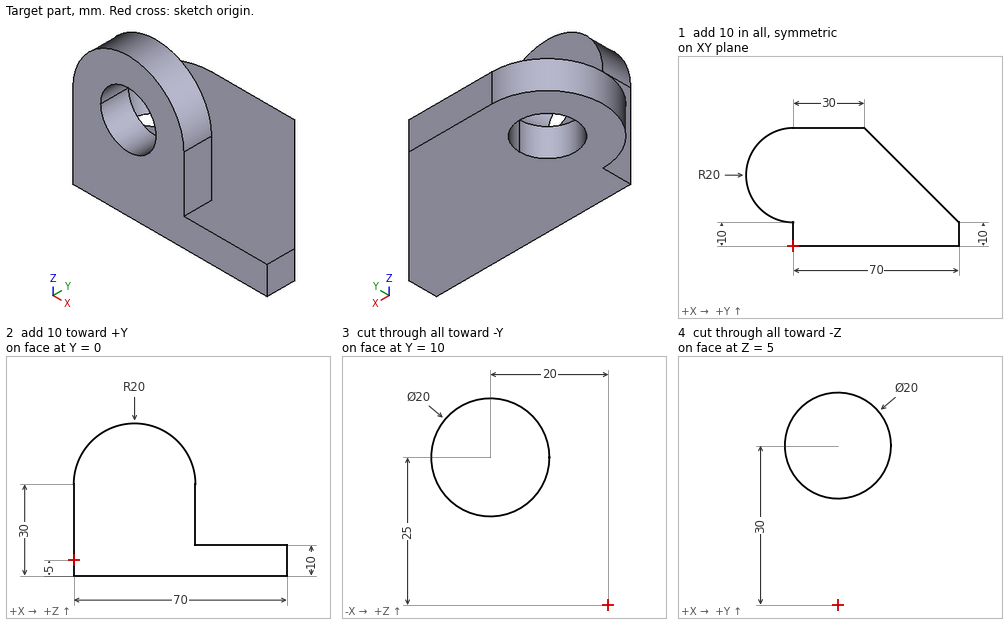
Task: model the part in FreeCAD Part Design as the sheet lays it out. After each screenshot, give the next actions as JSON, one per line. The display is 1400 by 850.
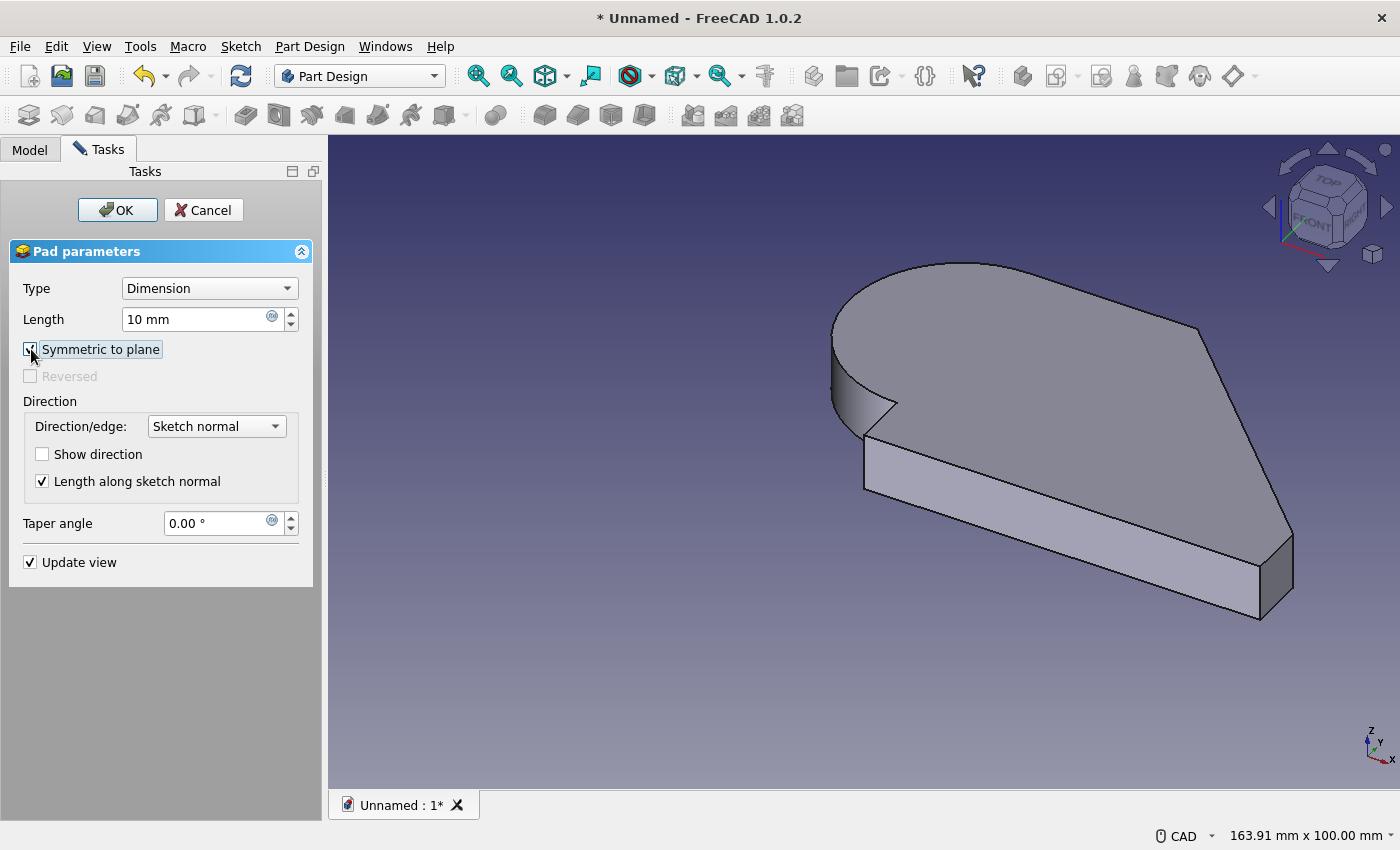
{"action": "left_click", "coordinate": [118, 210]}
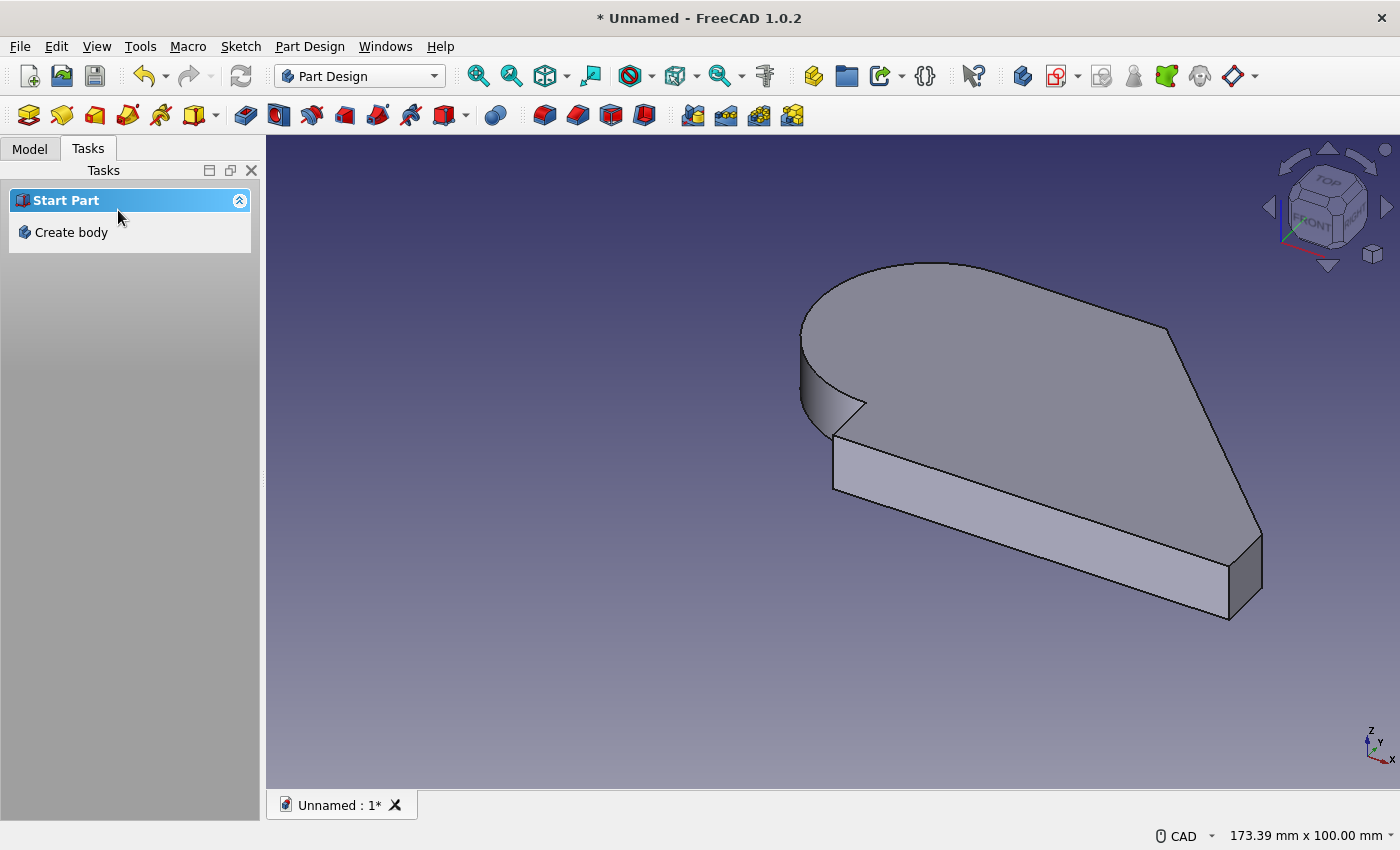
{"action": "left_click", "coordinate": [1201, 583]}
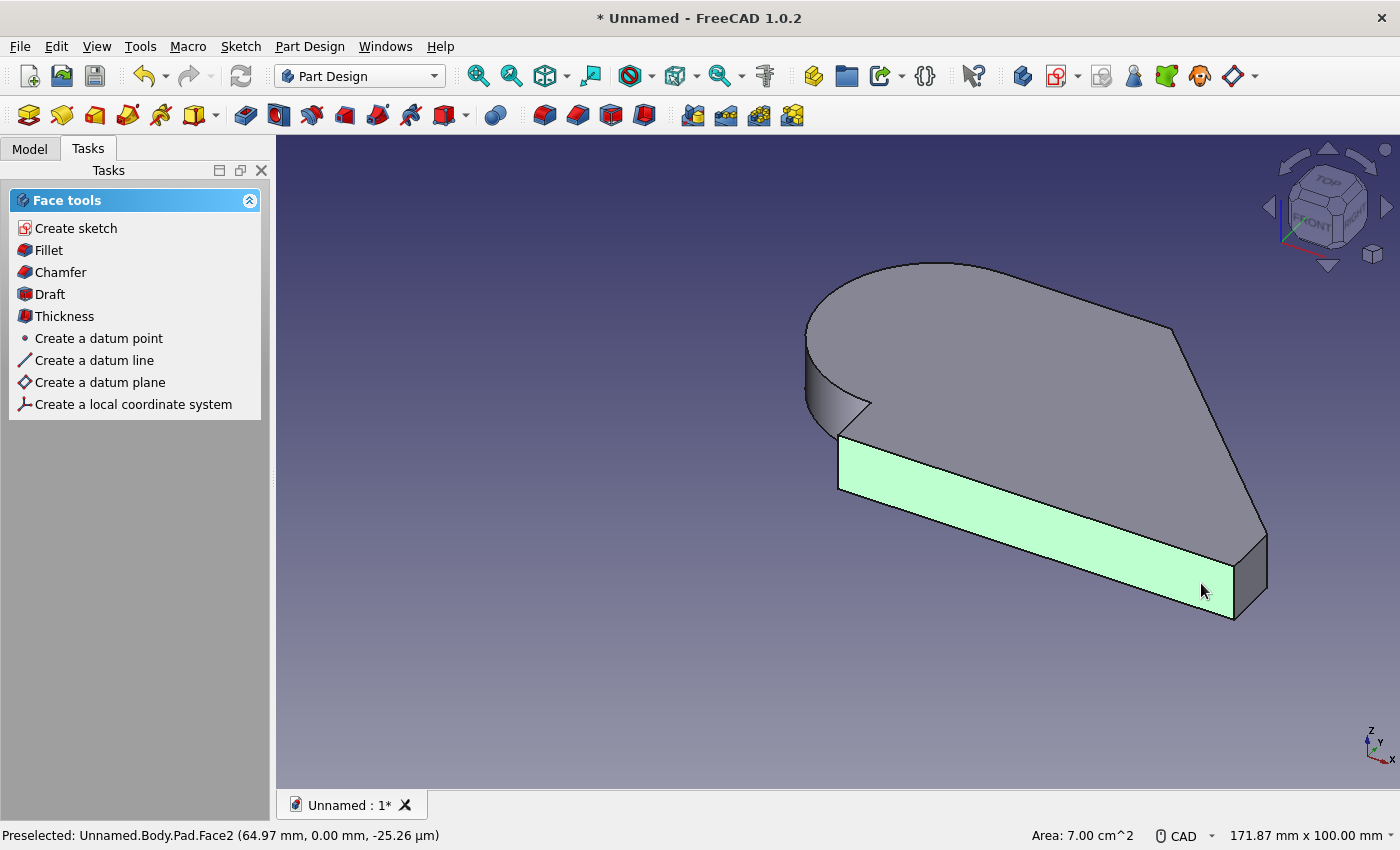
{"action": "left_click", "coordinate": [1056, 76]}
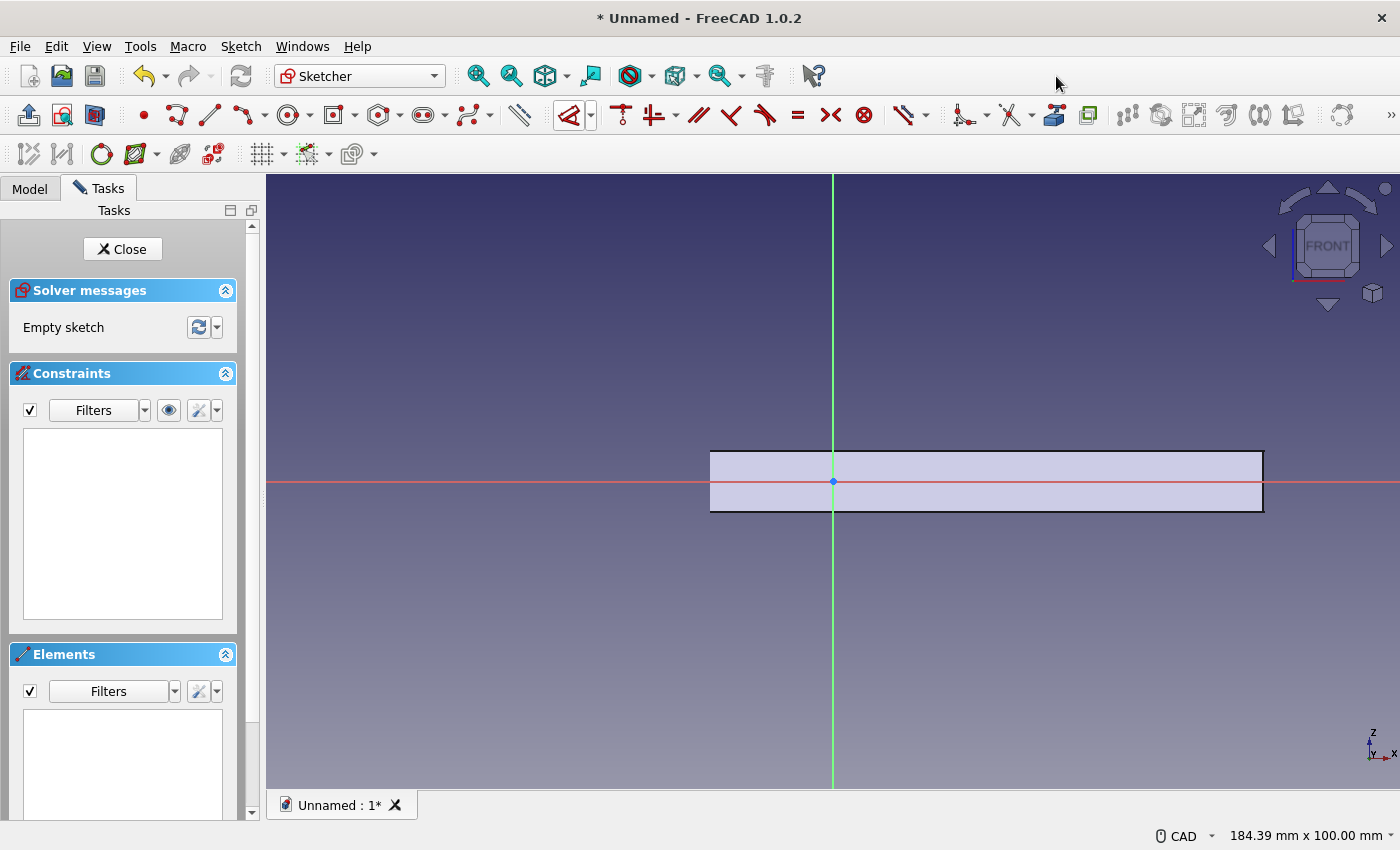
{"action": "scroll", "coordinate": [294, 761], "scroll_direction": "down", "scroll_amount": 1}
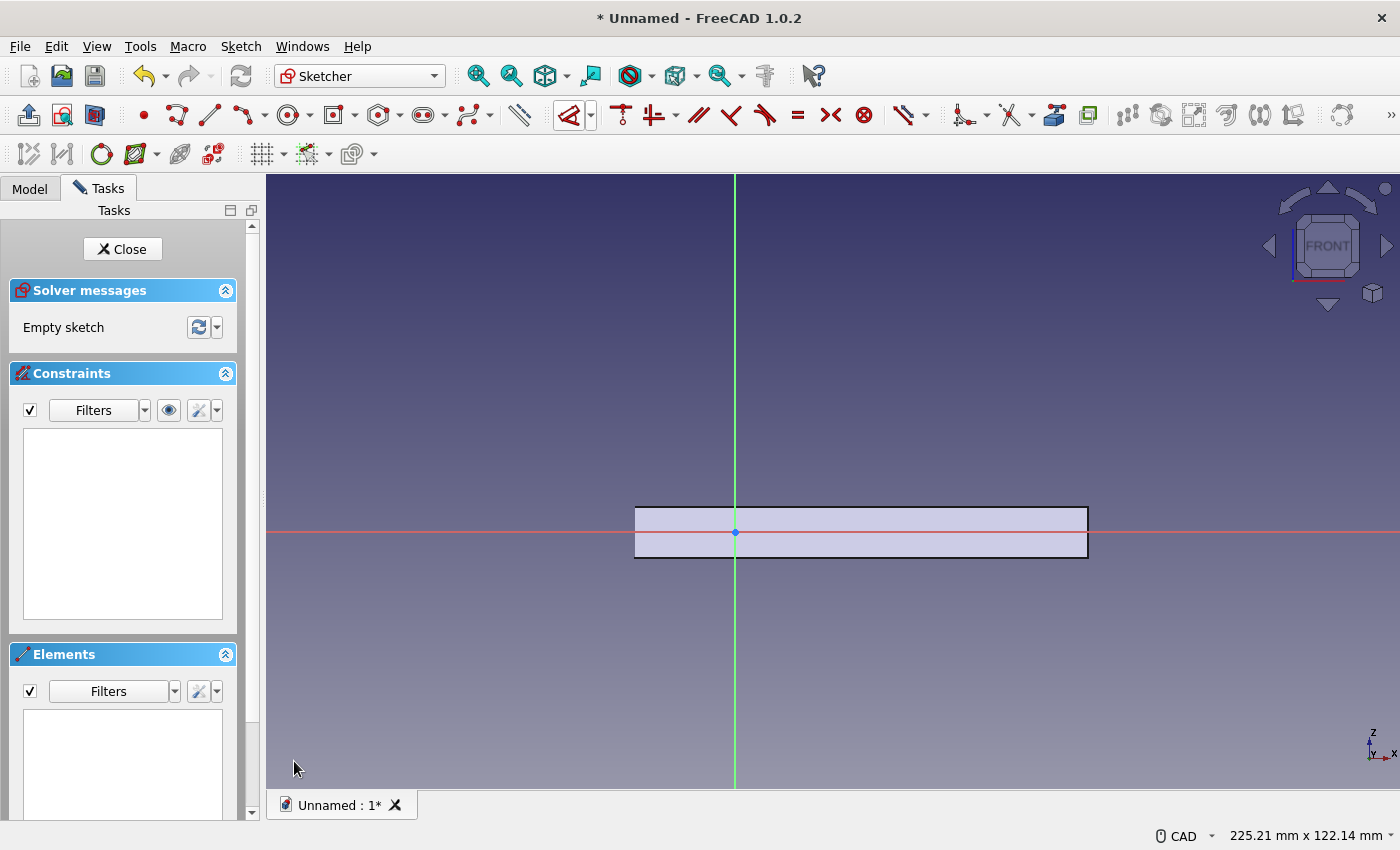
{"action": "scroll", "coordinate": [1210, 330], "scroll_direction": "up", "scroll_amount": 2}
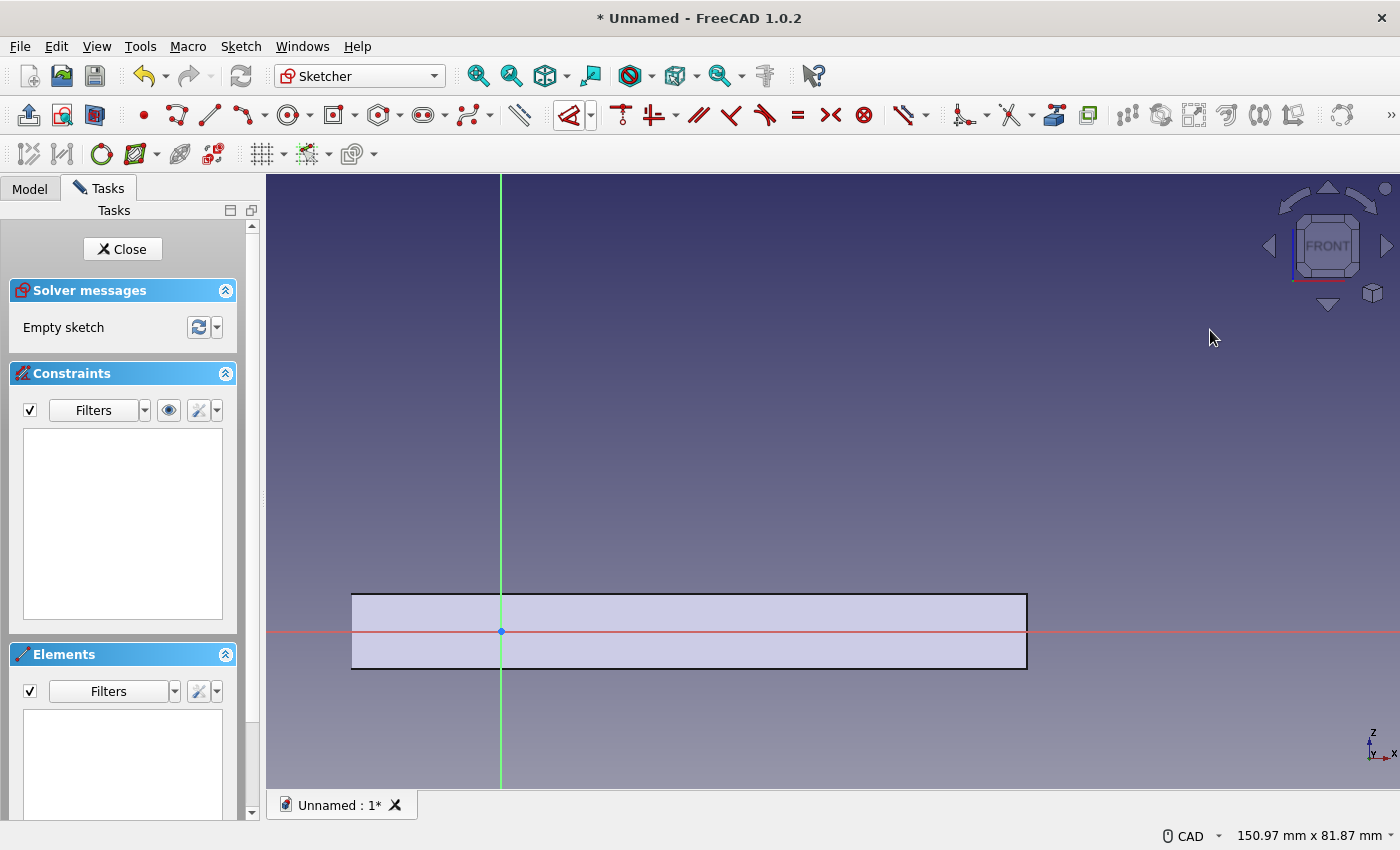
{"action": "left_click", "coordinate": [177, 116]}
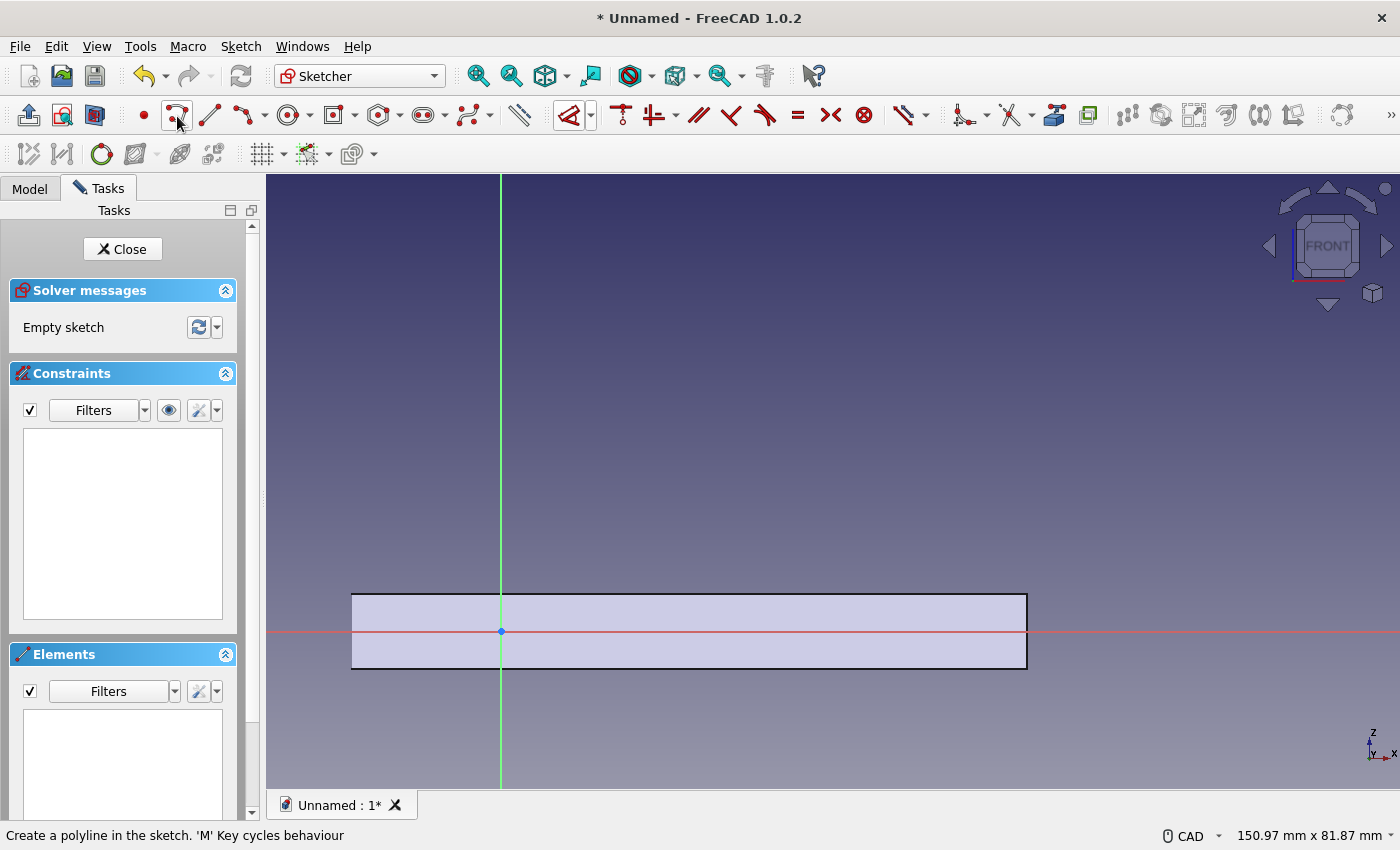
{"action": "left_click", "coordinate": [501, 444]}
{"action": "left_click", "coordinate": [510, 669]}
{"action": "left_click", "coordinate": [1027, 669]}
{"action": "left_click", "coordinate": [1027, 594]}
{"action": "left_click", "coordinate": [802, 594]}
{"action": "left_click", "coordinate": [802, 444]}
{"action": "right_click", "coordinate": [802, 444]}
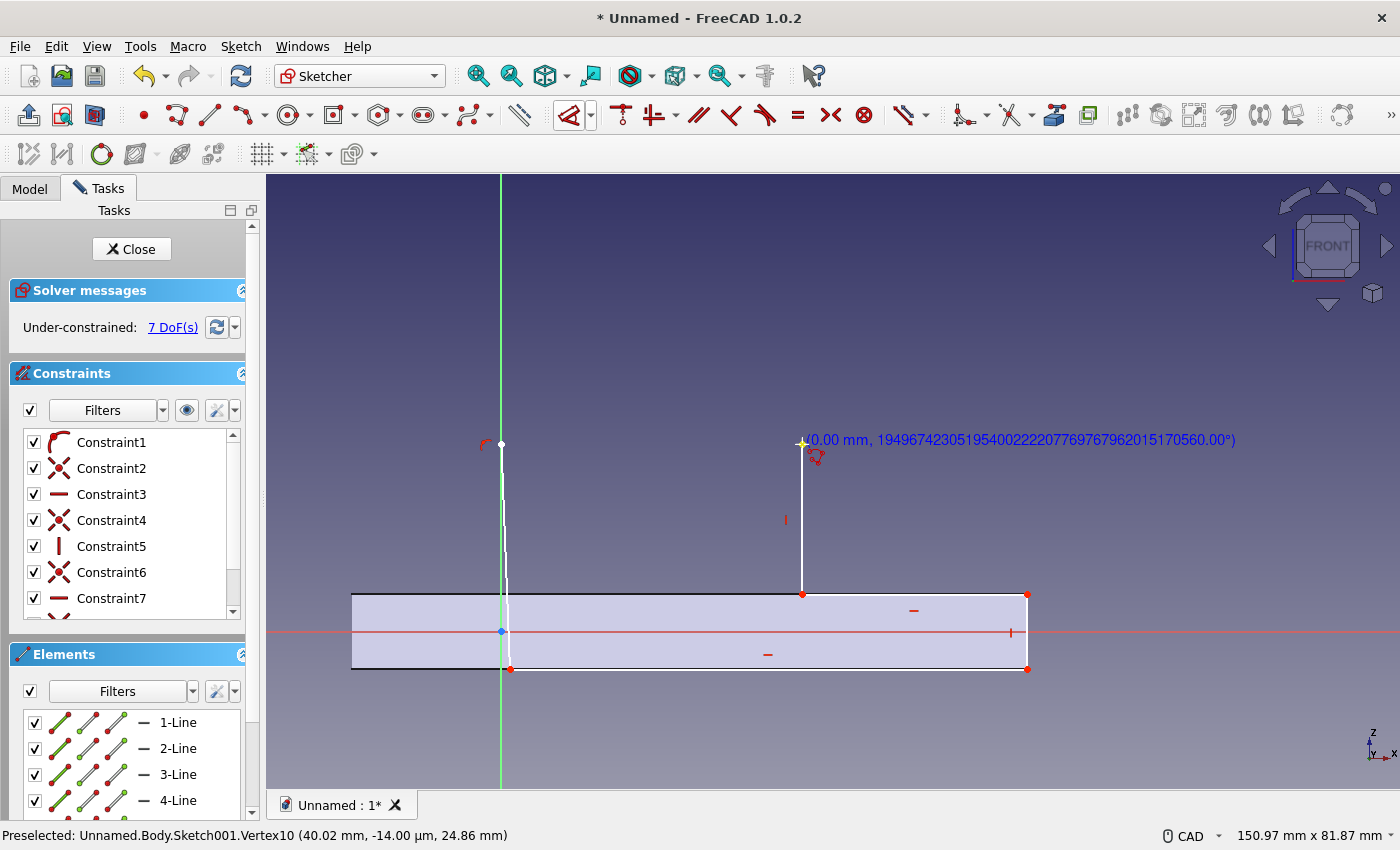
{"action": "left_click", "coordinate": [242, 116]}